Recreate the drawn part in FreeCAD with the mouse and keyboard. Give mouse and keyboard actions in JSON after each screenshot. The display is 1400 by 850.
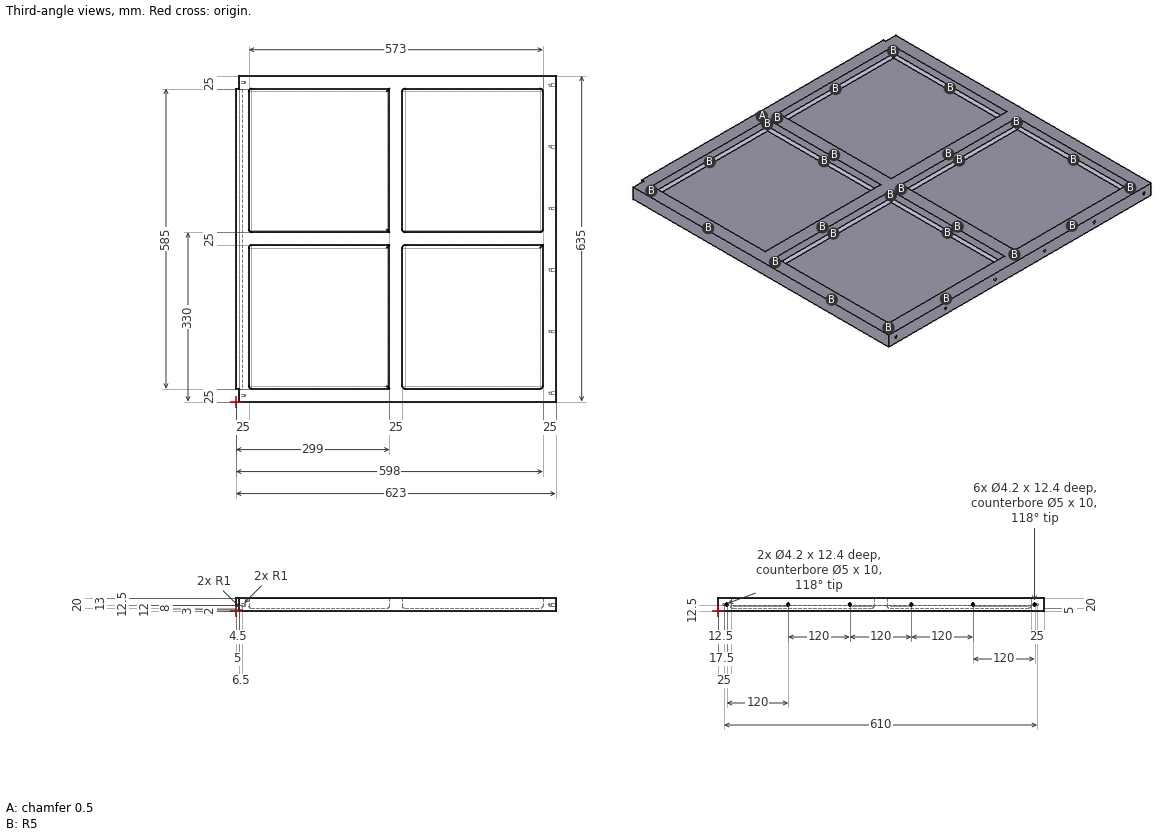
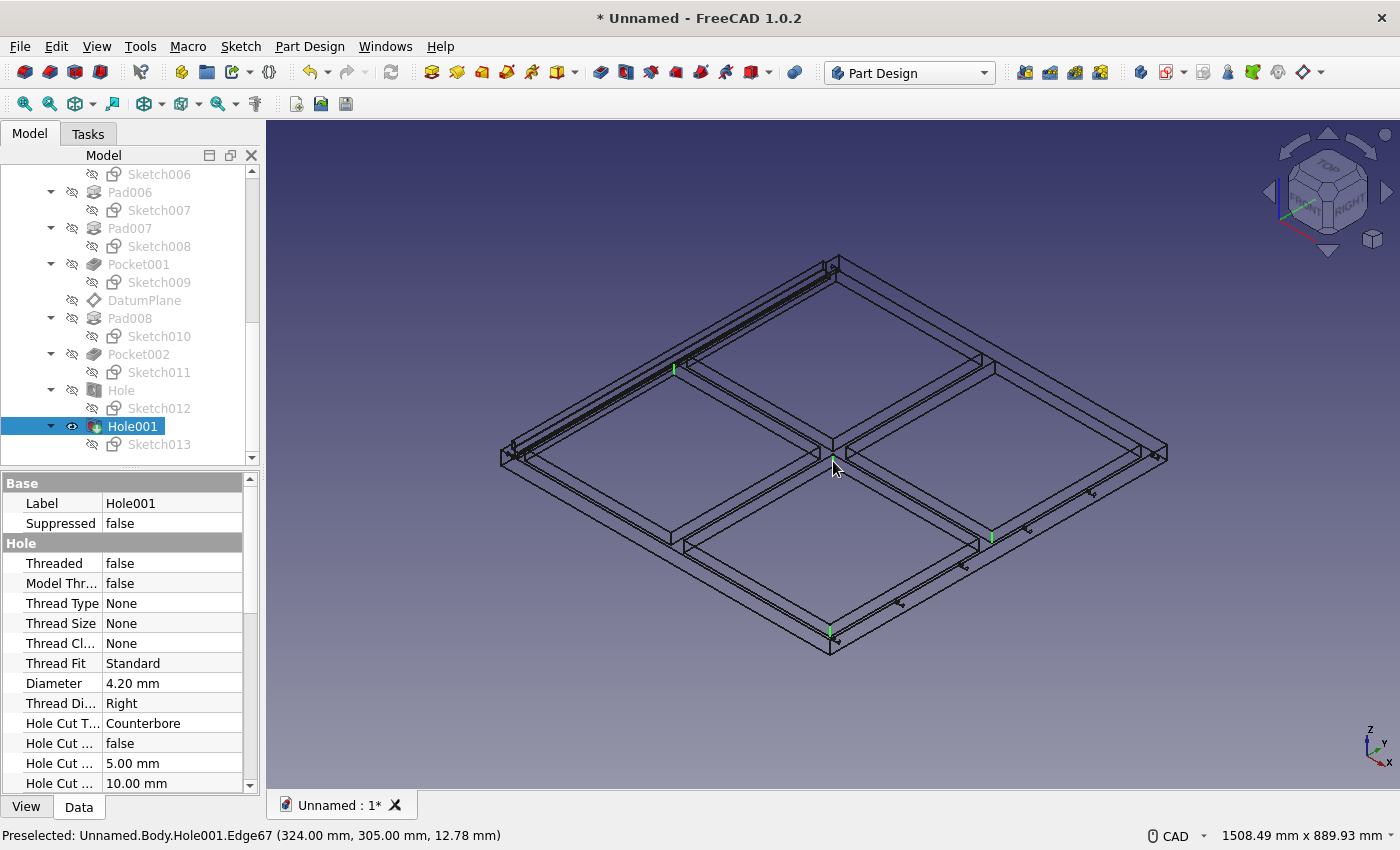
{"action": "left_click", "coordinate": [684, 547], "text": "ctrl"}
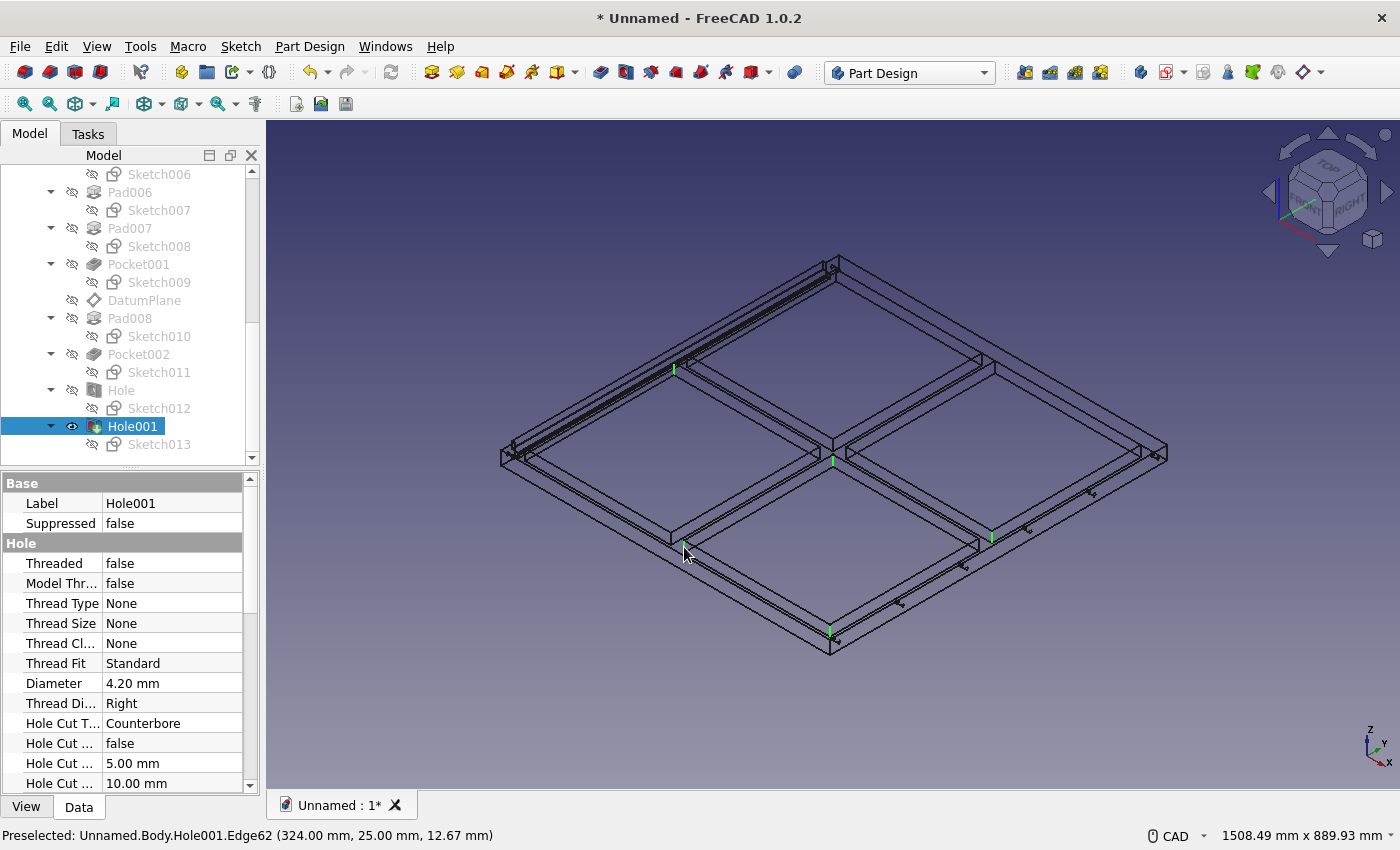
{"action": "left_click", "coordinate": [995, 368], "text": "ctrl"}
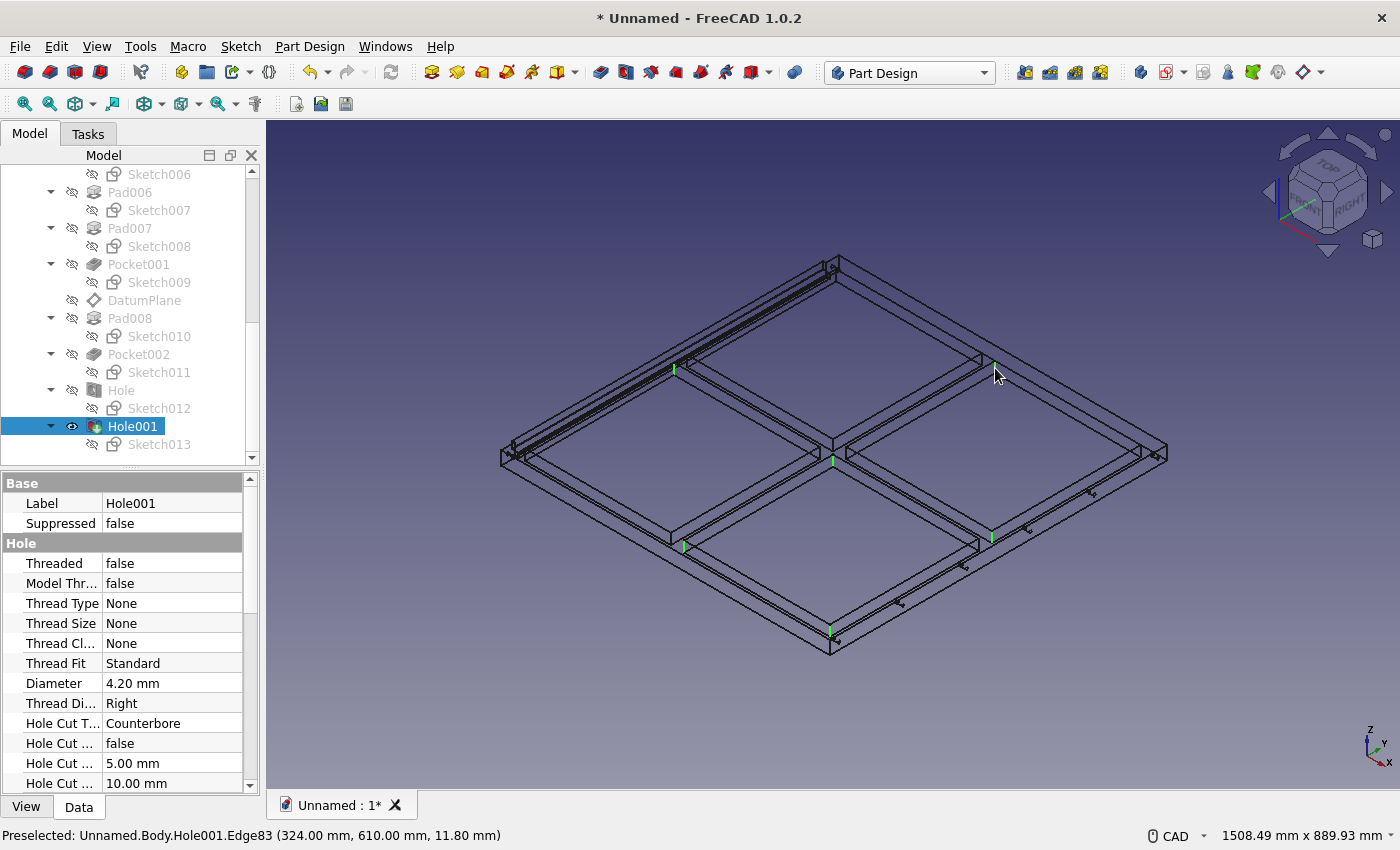
{"action": "left_click", "coordinate": [836, 277], "text": "ctrl"}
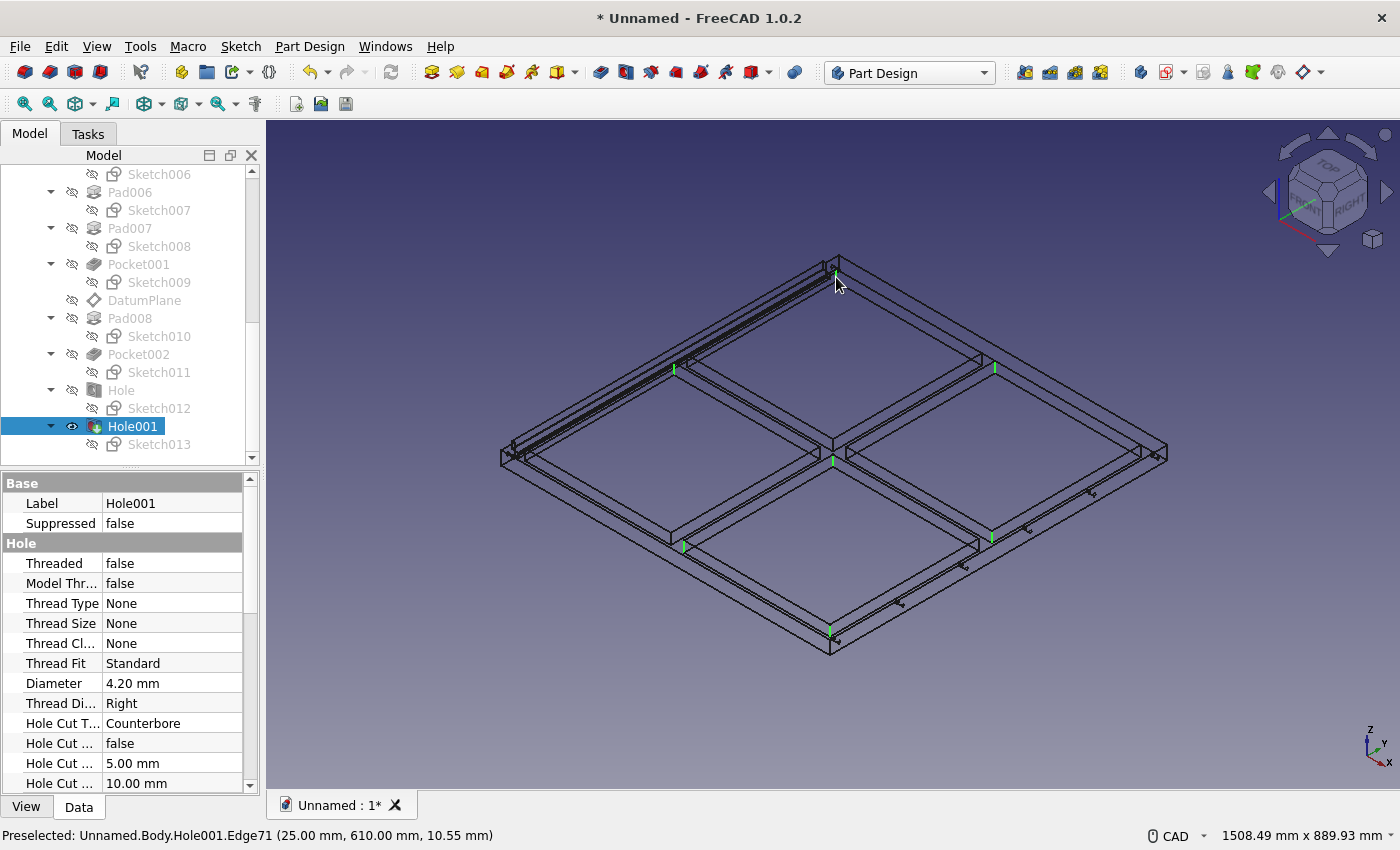
{"action": "left_click", "coordinate": [525, 455], "text": "ctrl"}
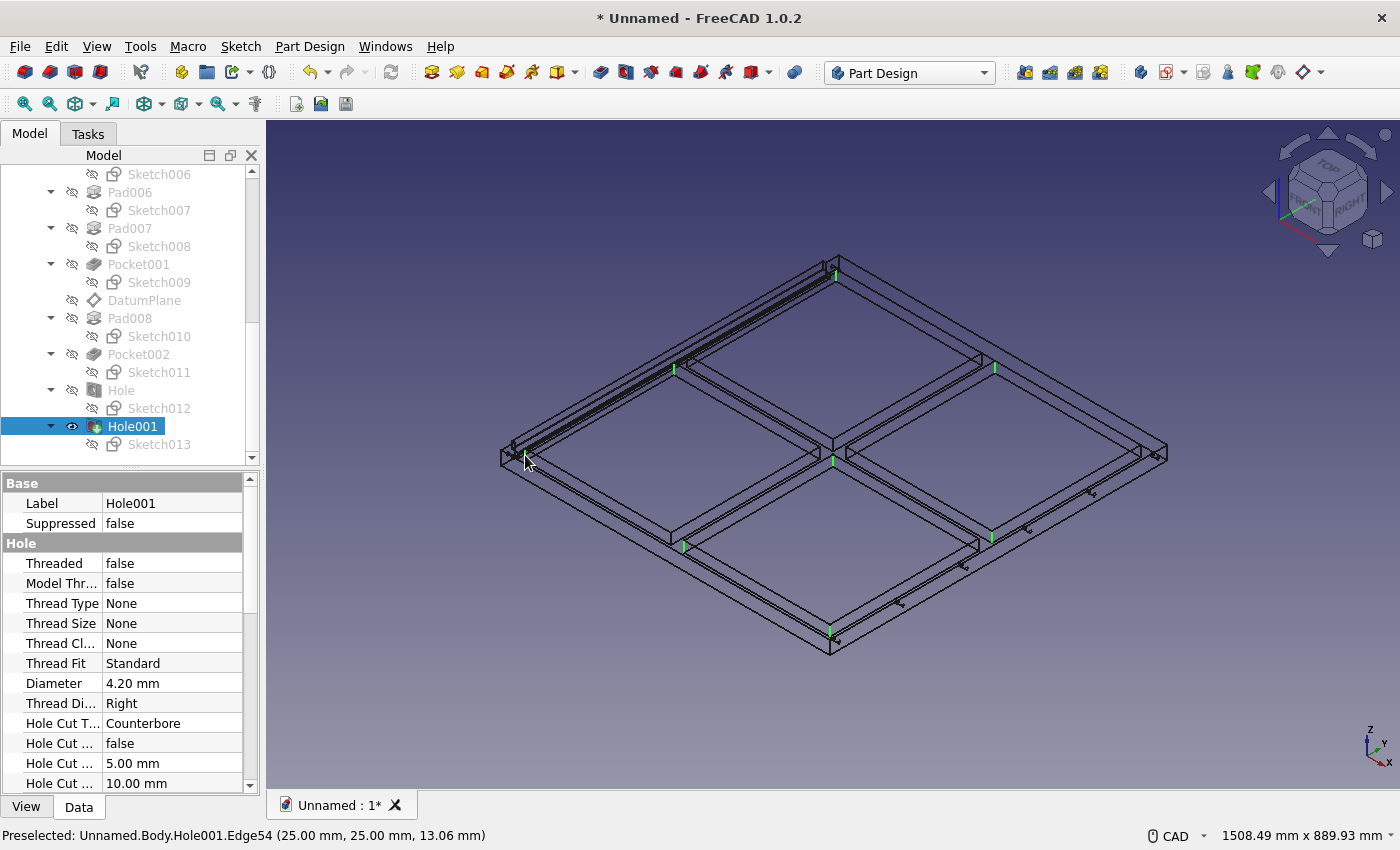
{"action": "scroll", "coordinate": [687, 360], "scroll_direction": "up", "scroll_amount": 6}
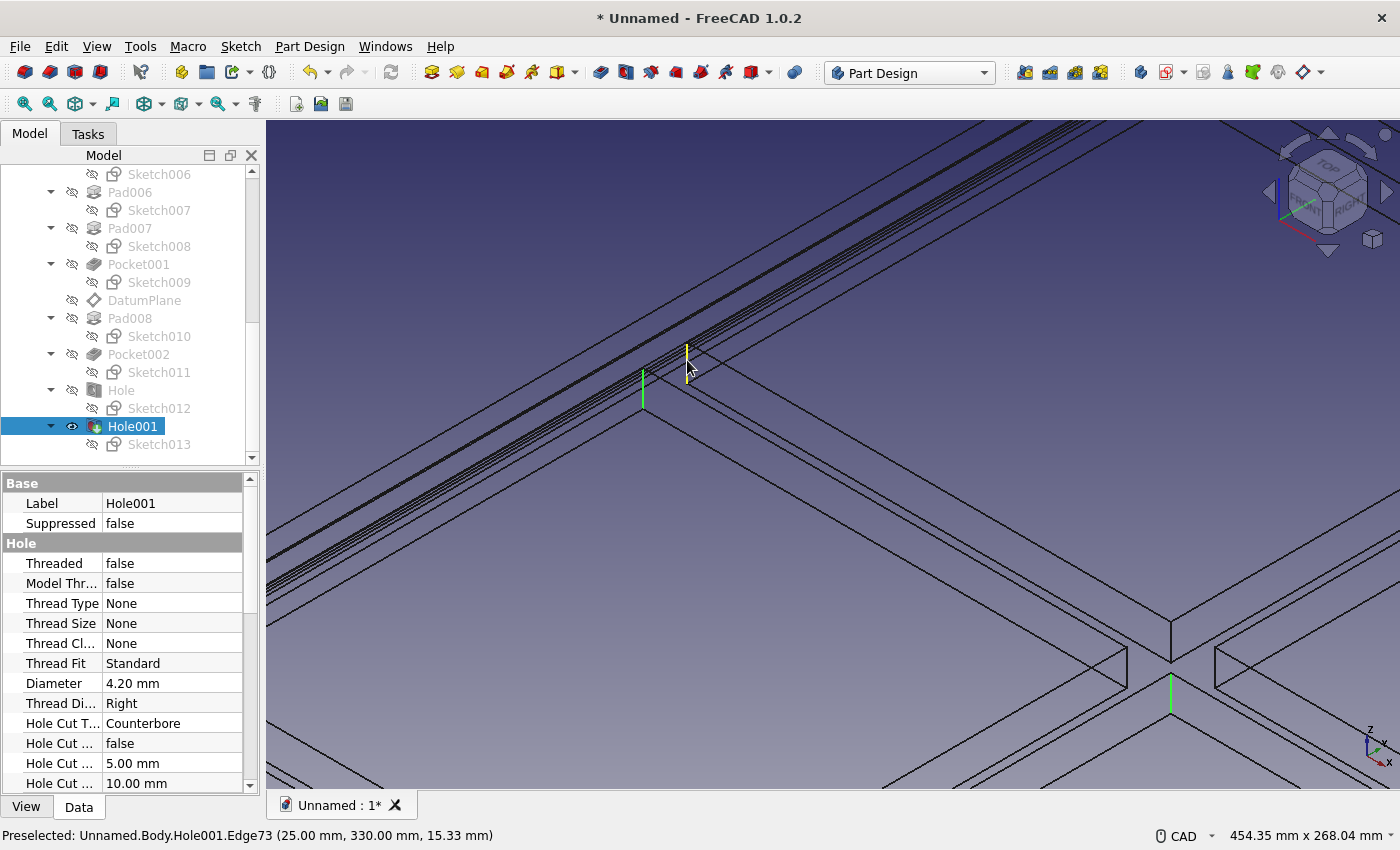
{"action": "left_click", "coordinate": [687, 362], "text": "ctrl"}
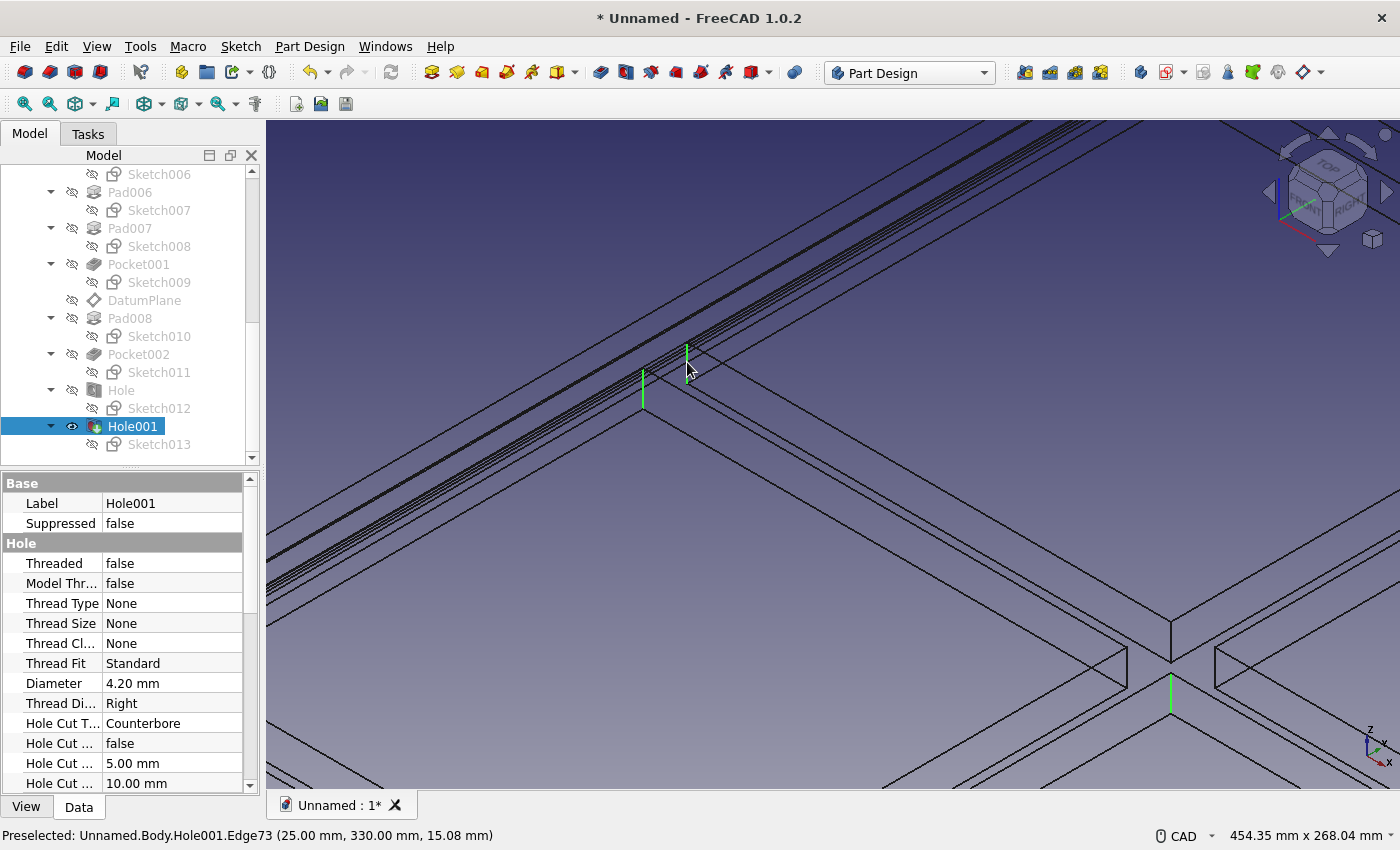
{"action": "left_click", "coordinate": [1215, 667], "text": "ctrl"}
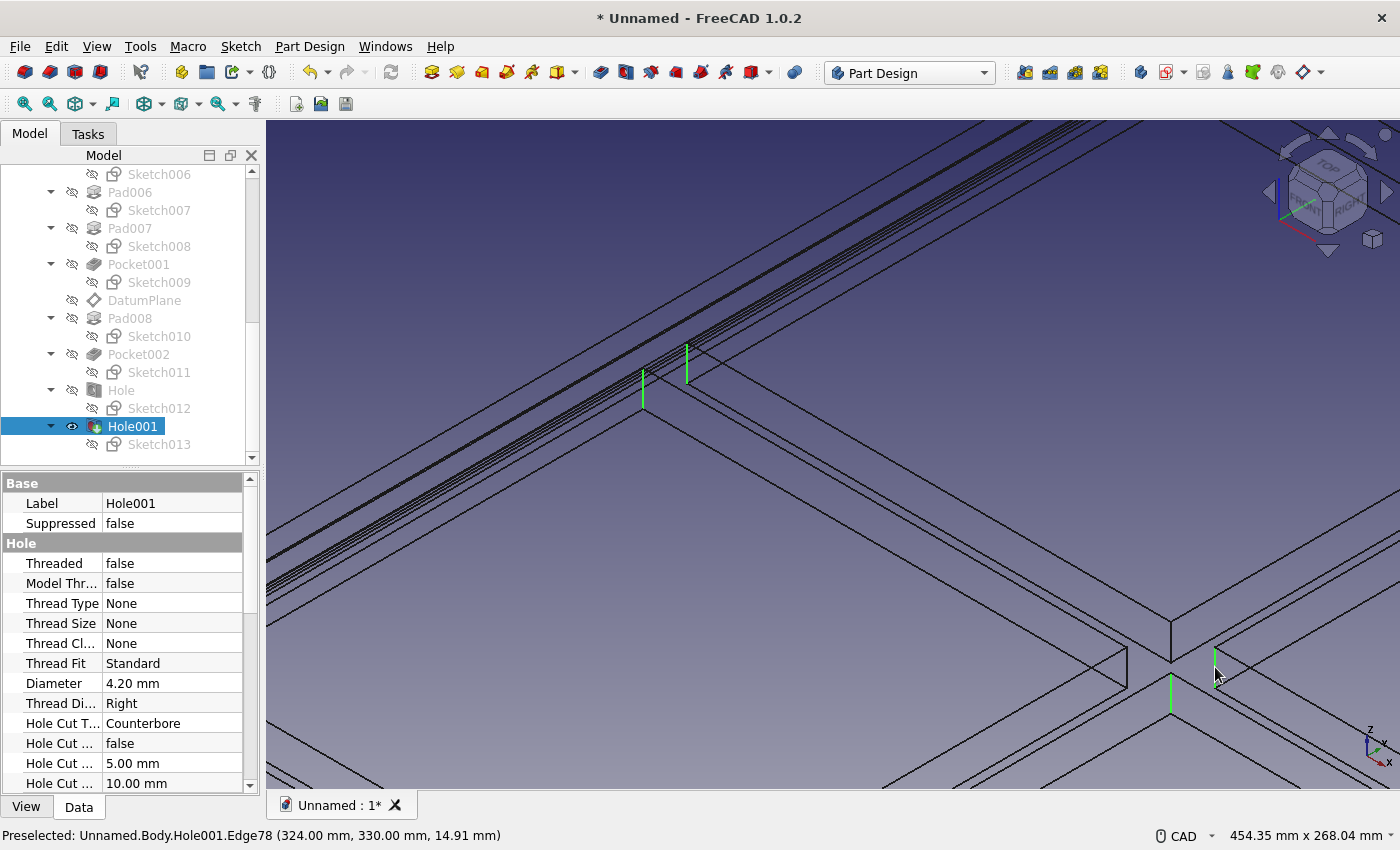
{"action": "left_click", "coordinate": [25, 104]}